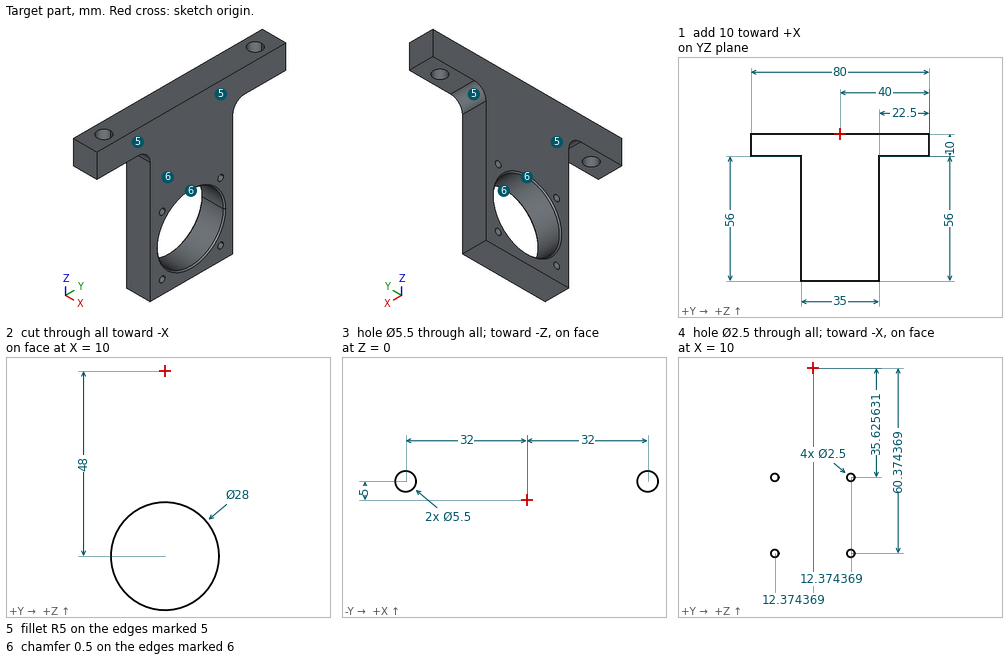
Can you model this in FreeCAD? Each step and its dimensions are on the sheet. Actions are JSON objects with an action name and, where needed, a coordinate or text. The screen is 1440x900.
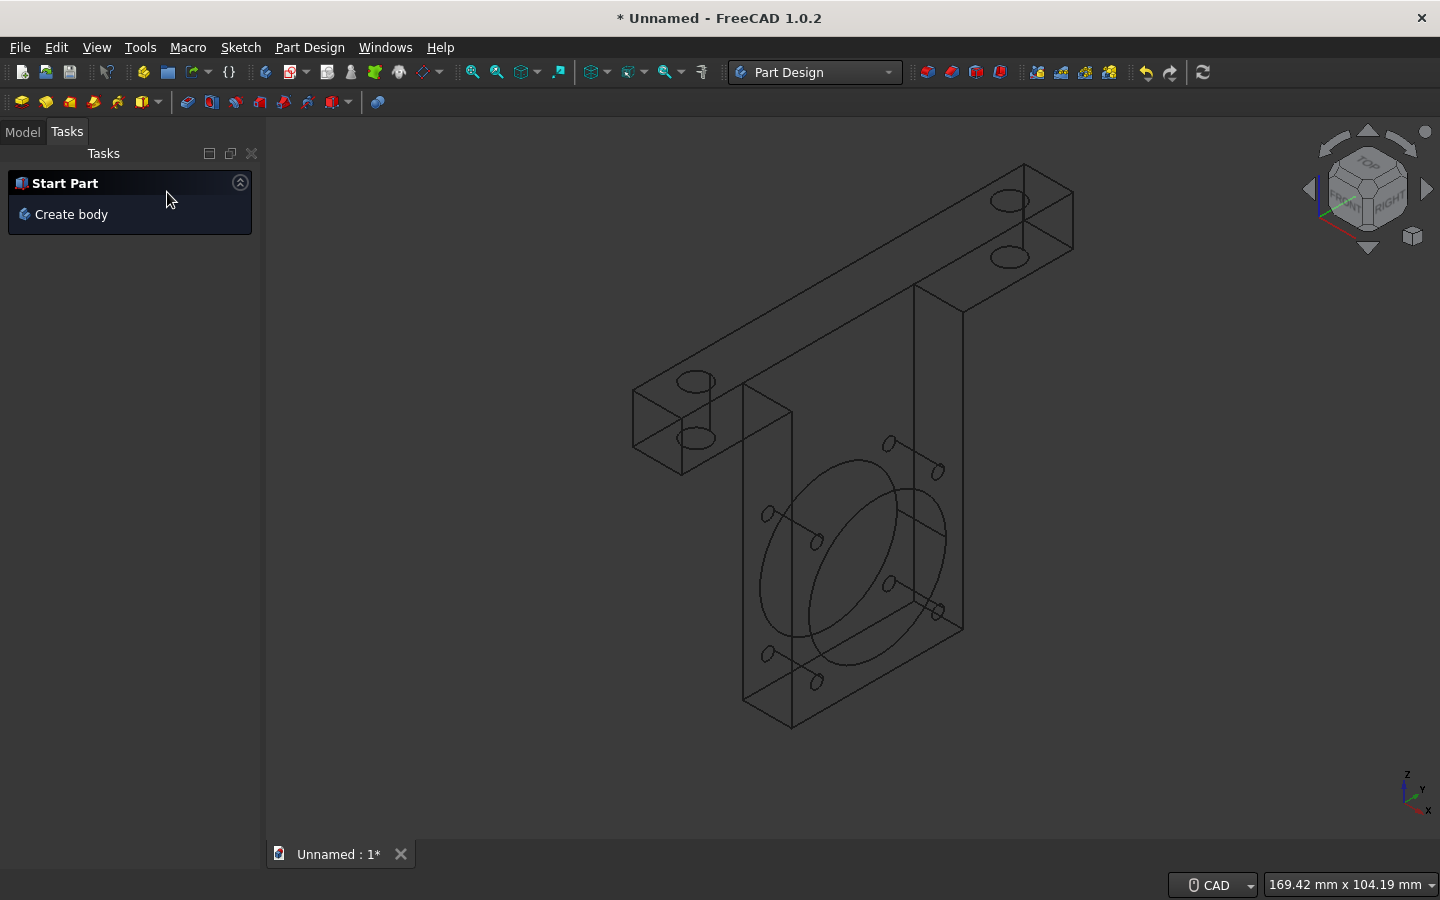
{"action": "left_click", "coordinate": [939, 297]}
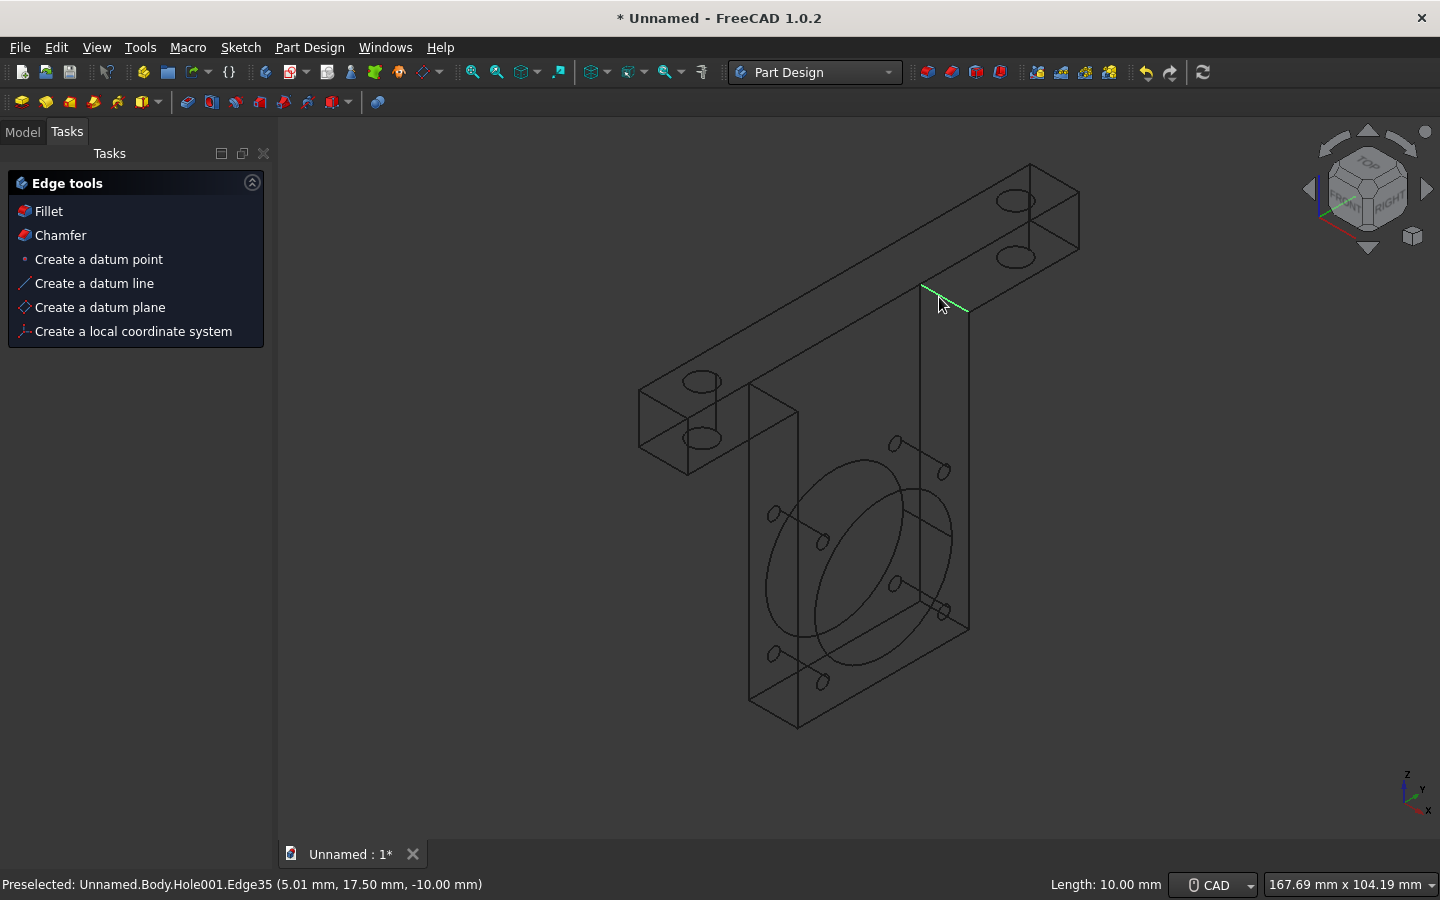
{"action": "left_click", "coordinate": [773, 396], "text": "ctrl"}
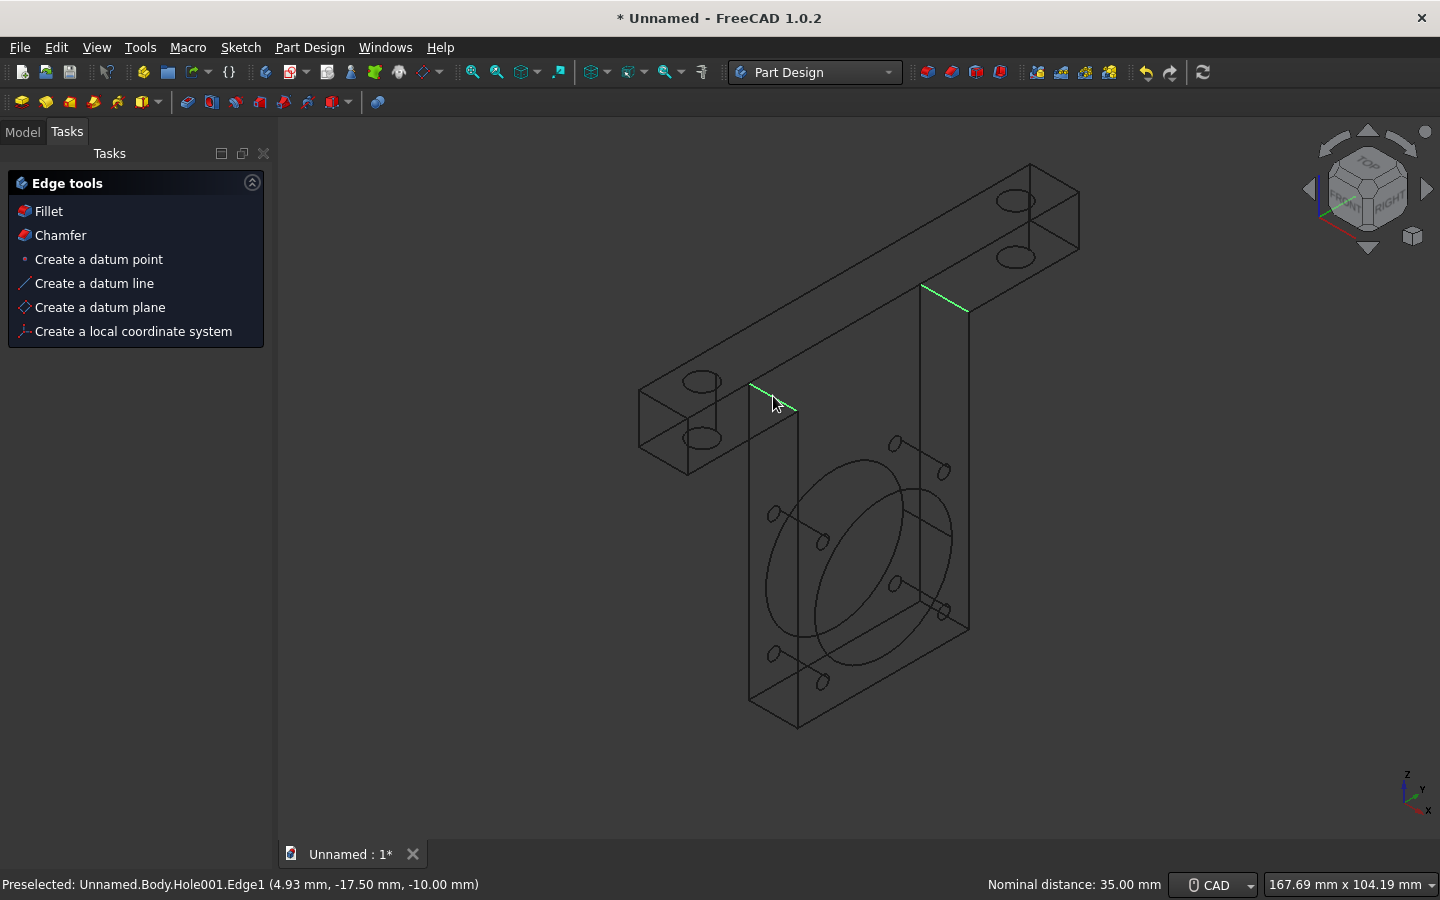
{"action": "key", "text": "v 1"}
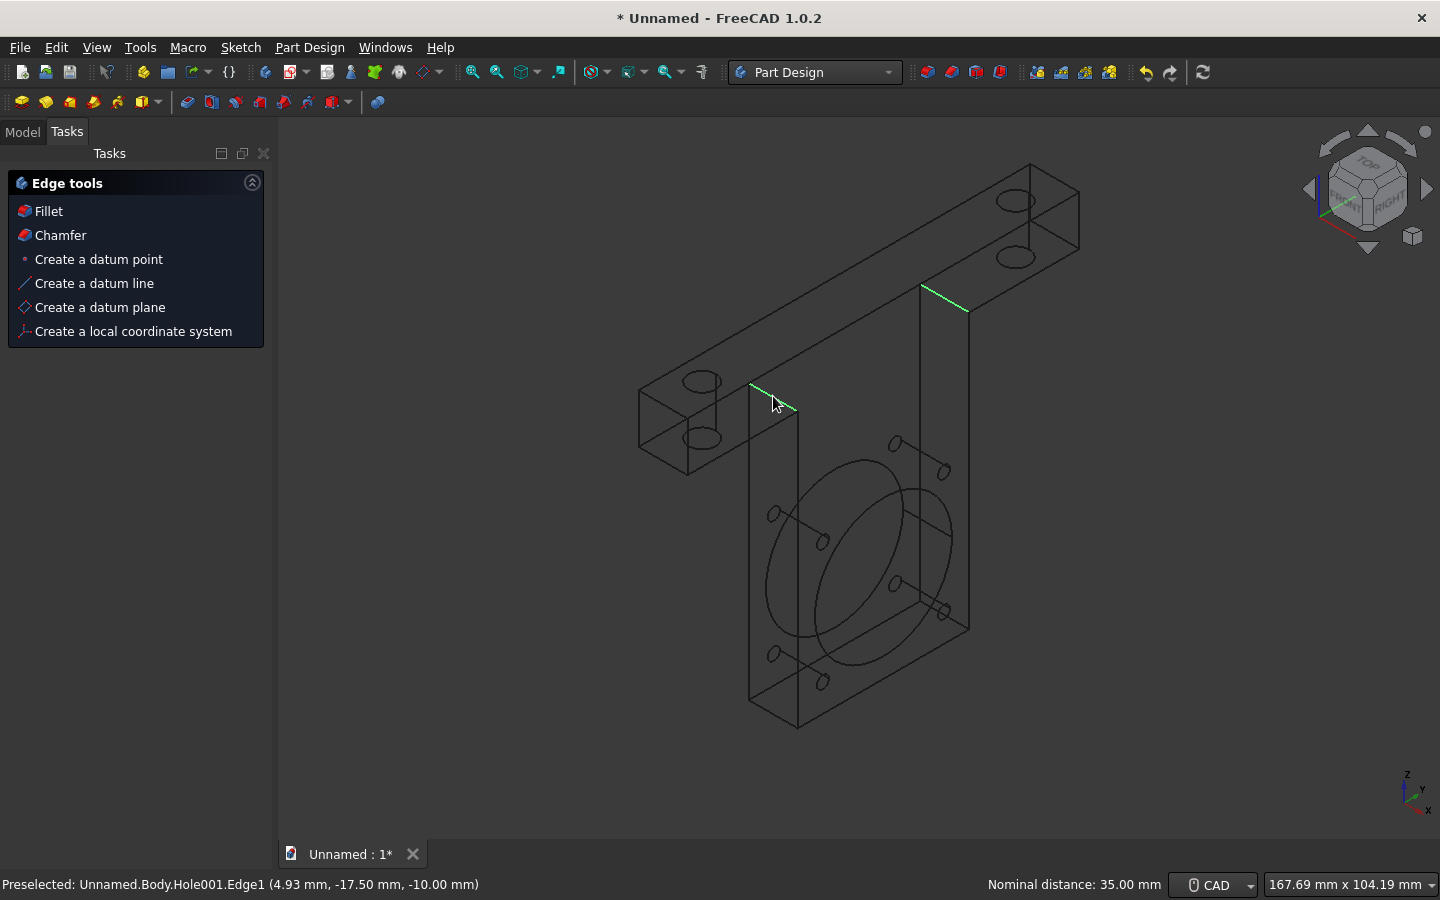
{"action": "left_click", "coordinate": [928, 72]}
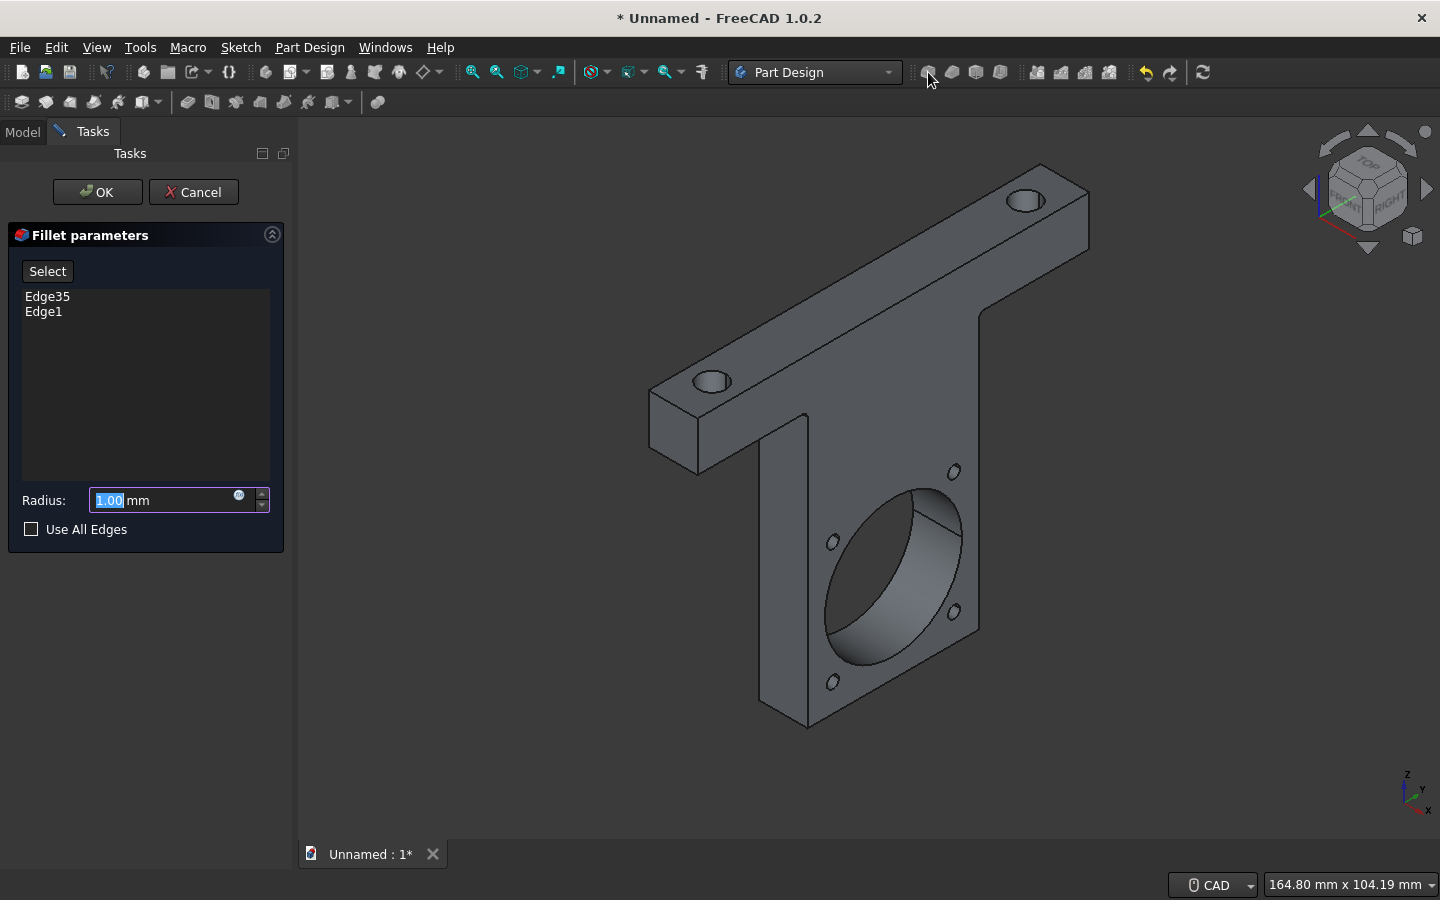
{"action": "type", "text": "5"}
{"action": "key", "text": "Tab"}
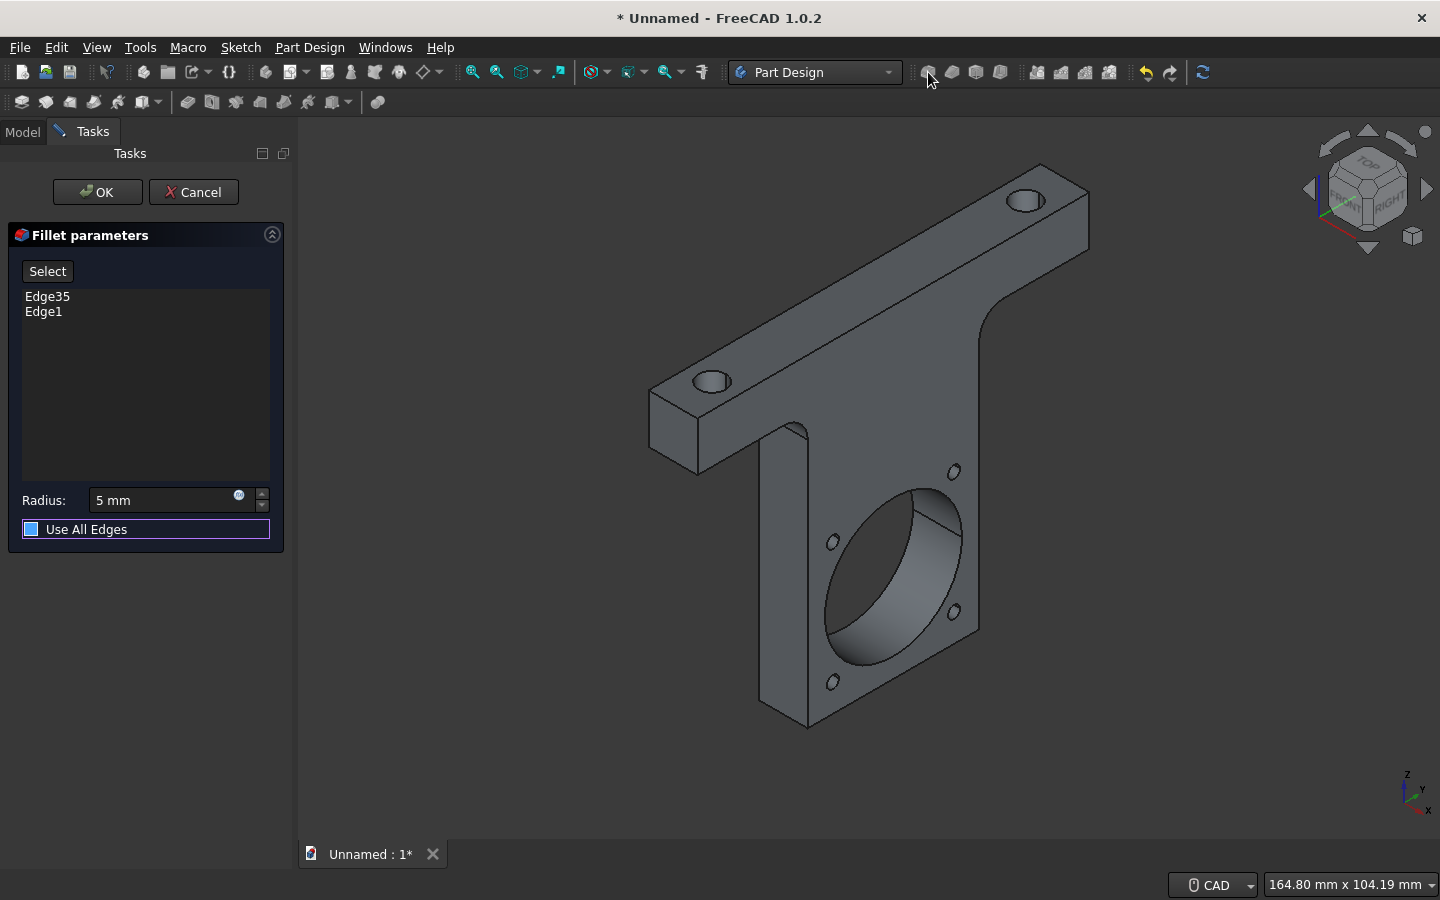
{"action": "left_click", "coordinate": [98, 192]}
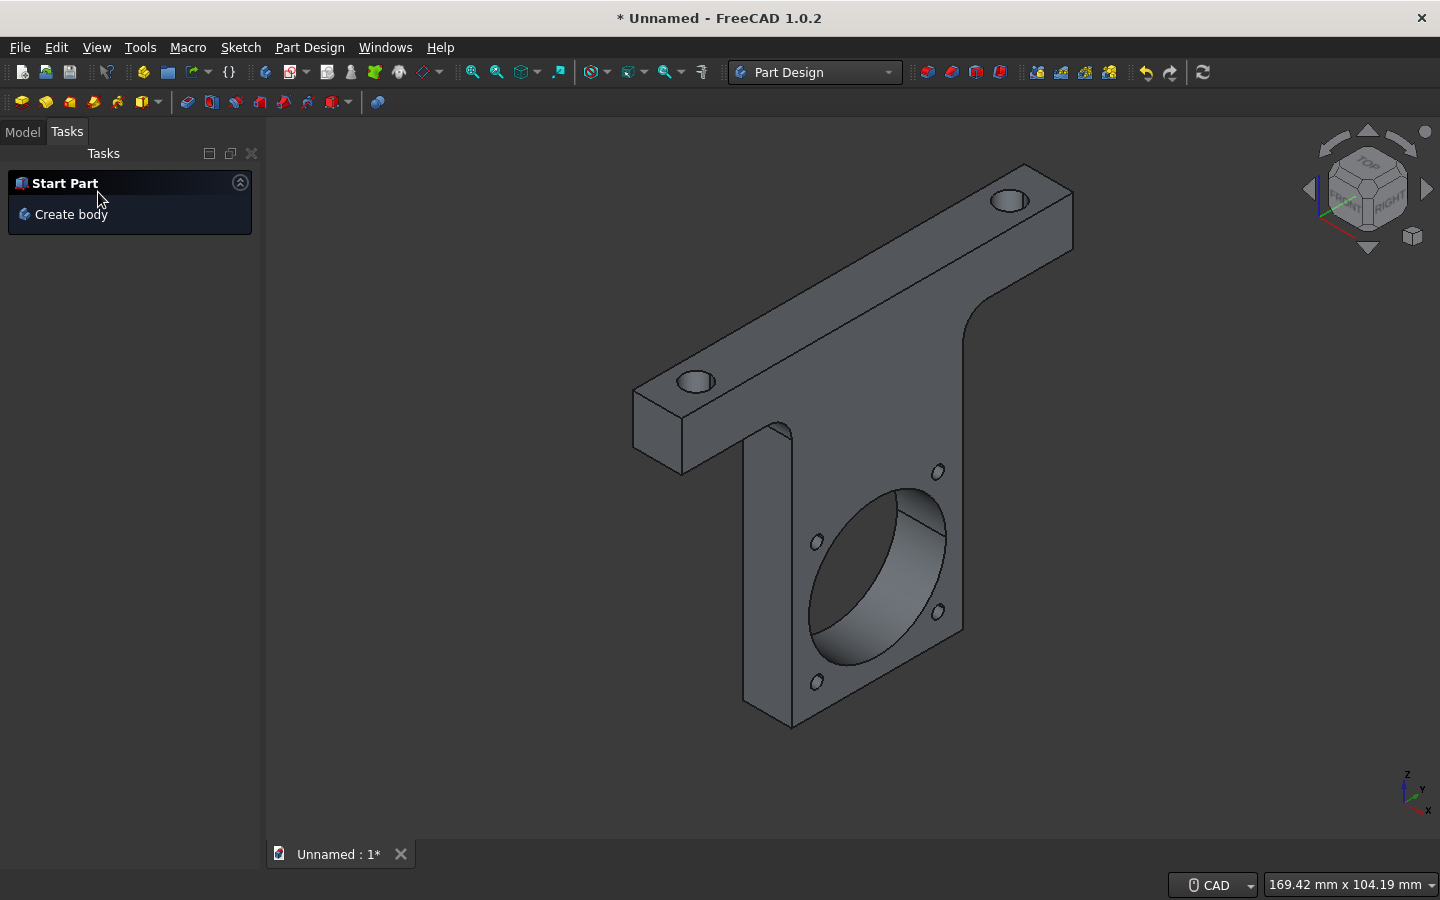
{"action": "left_click", "coordinate": [856, 664]}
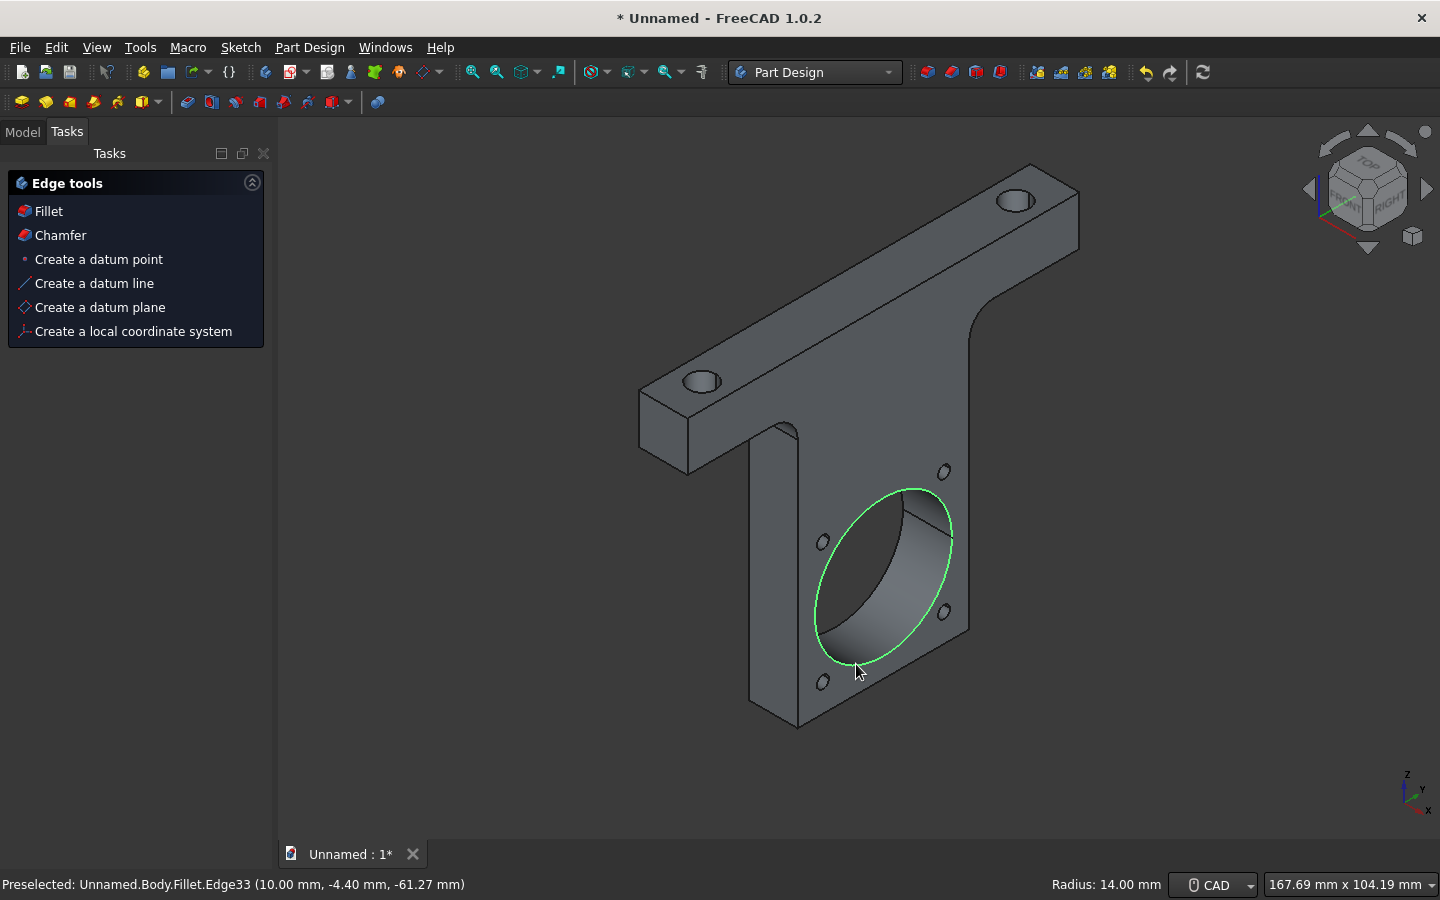
{"action": "key", "text": "2"}